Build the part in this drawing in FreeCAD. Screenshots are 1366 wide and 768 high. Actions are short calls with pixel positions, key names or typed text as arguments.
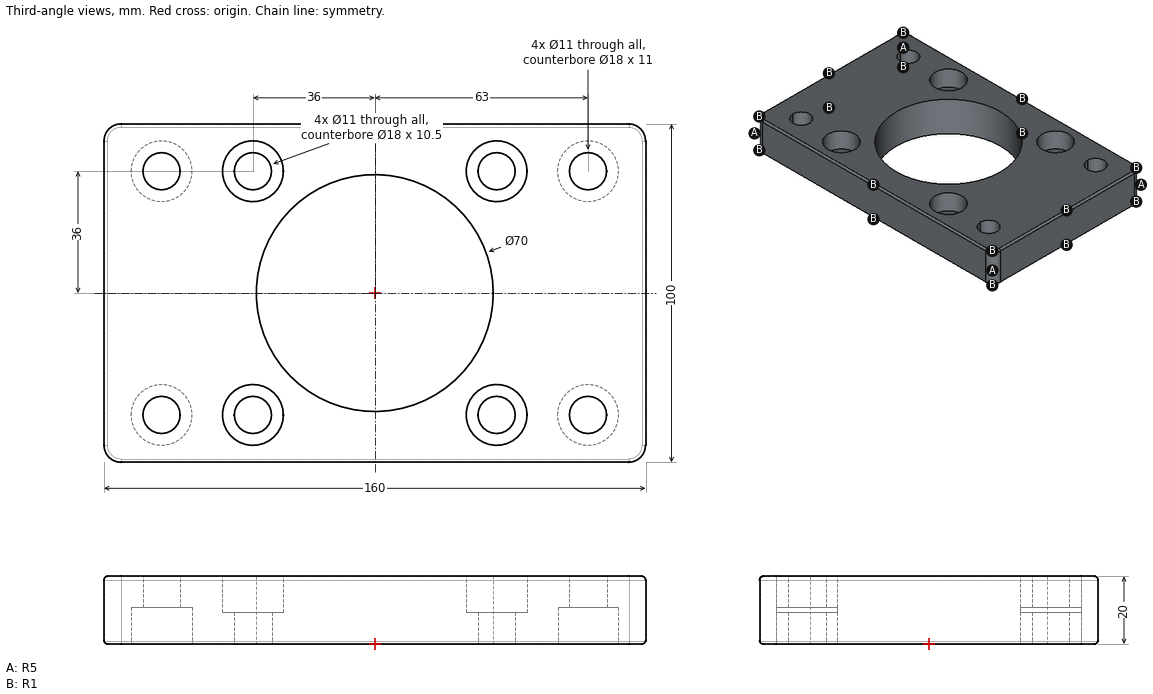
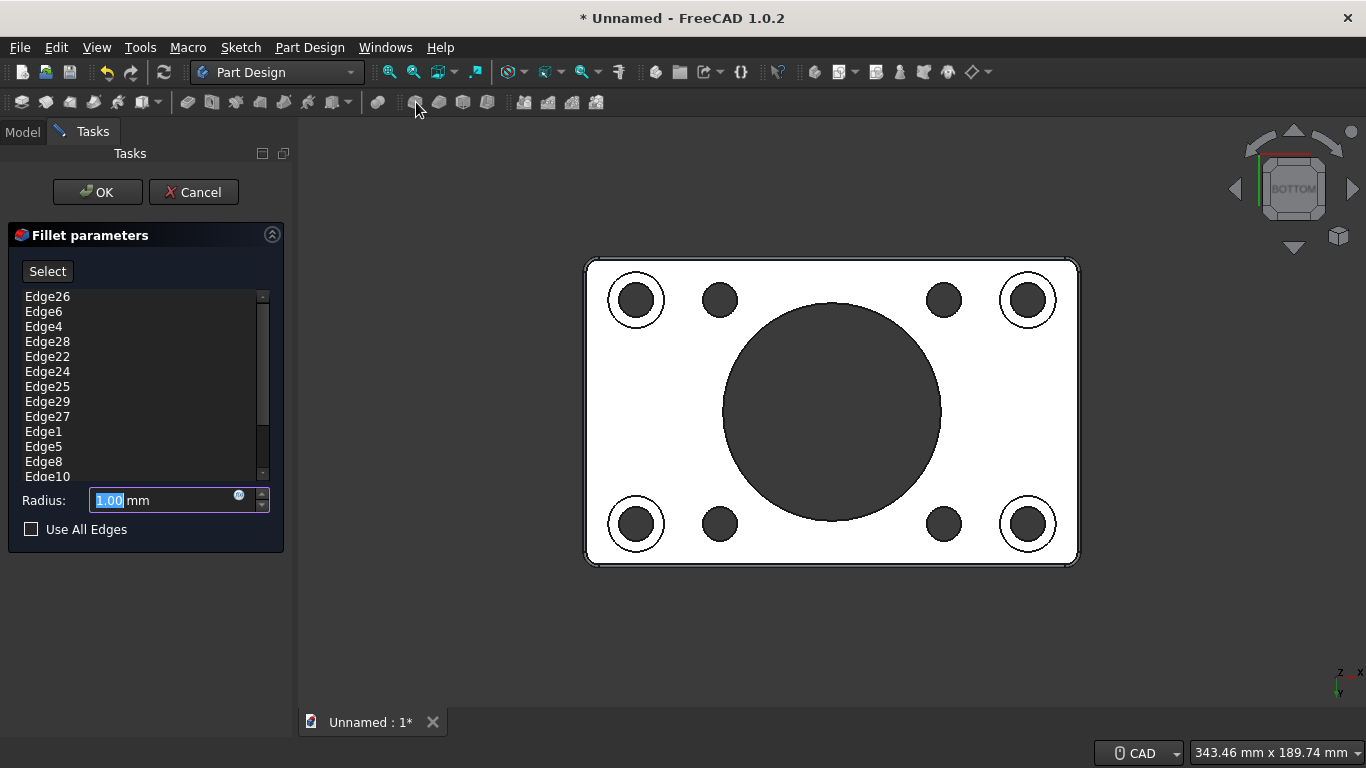
text(1)
key(Tab)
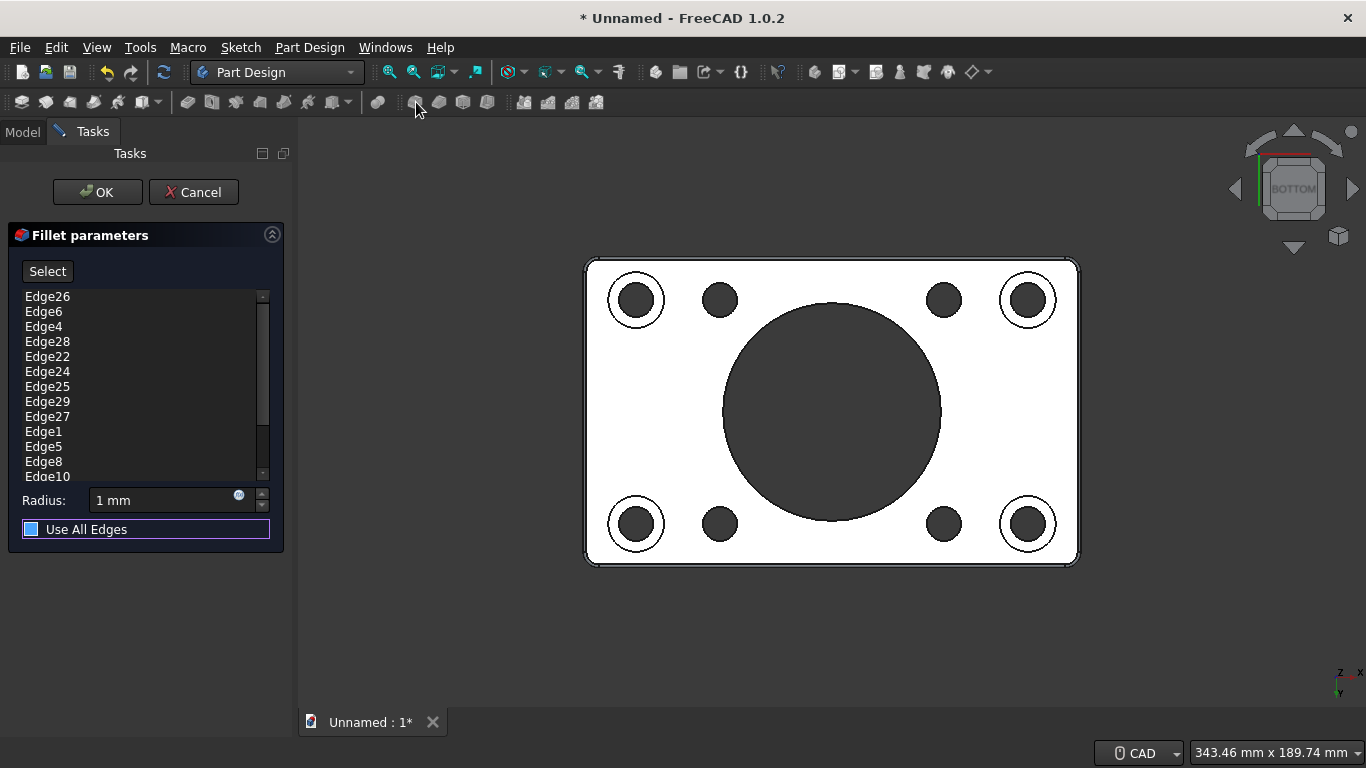
click(98, 192)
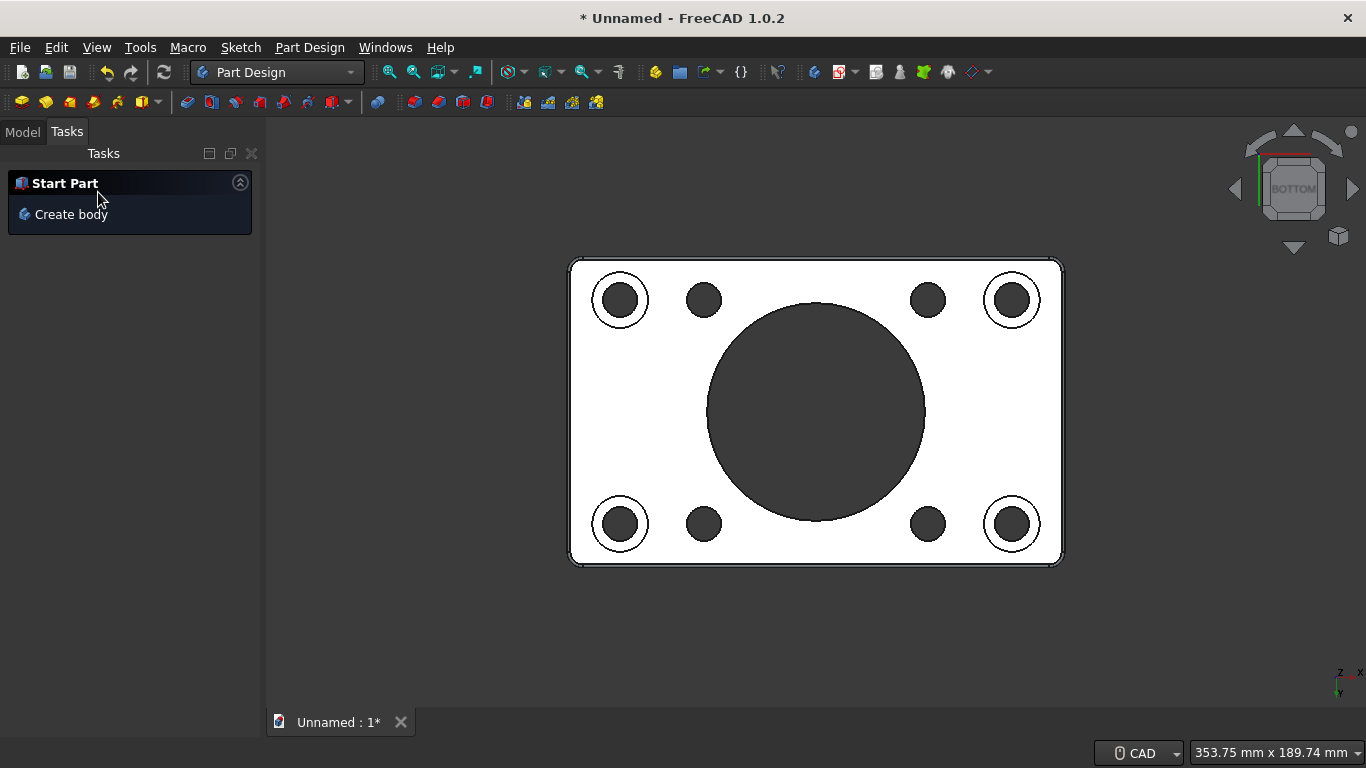
key(0)